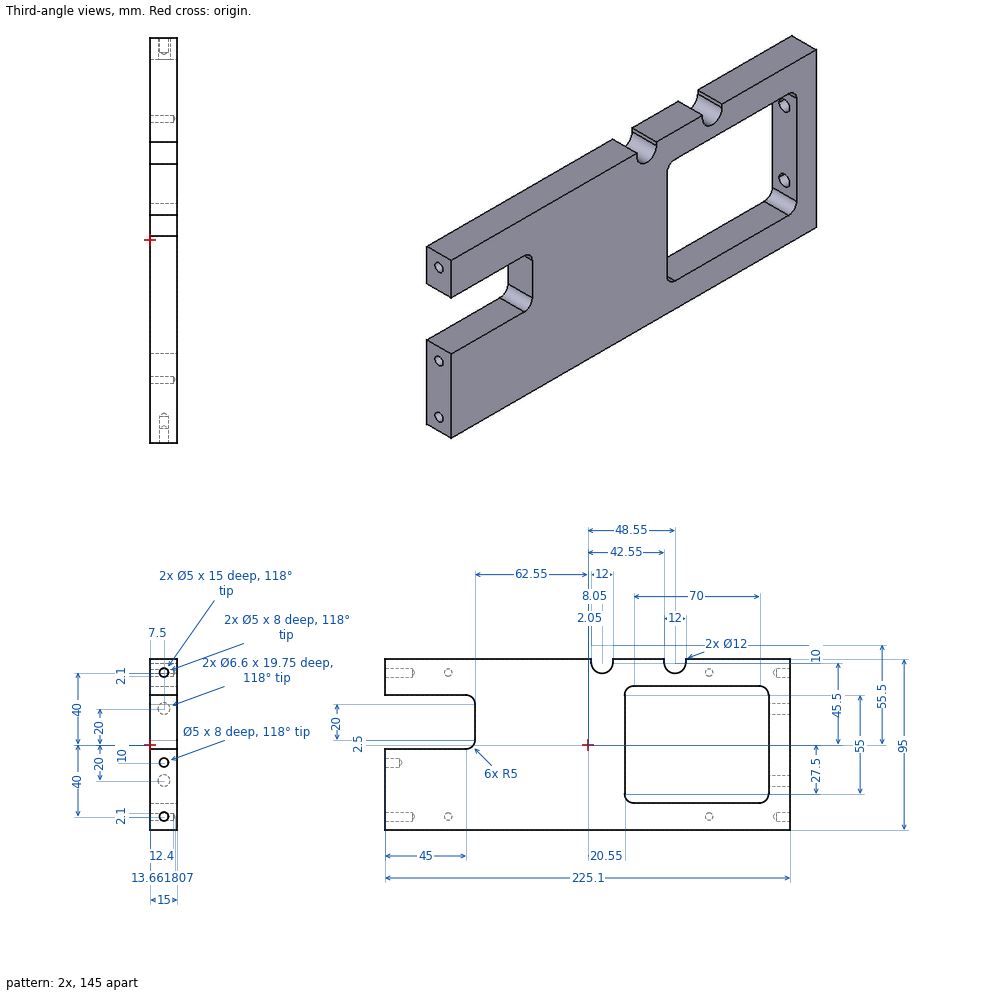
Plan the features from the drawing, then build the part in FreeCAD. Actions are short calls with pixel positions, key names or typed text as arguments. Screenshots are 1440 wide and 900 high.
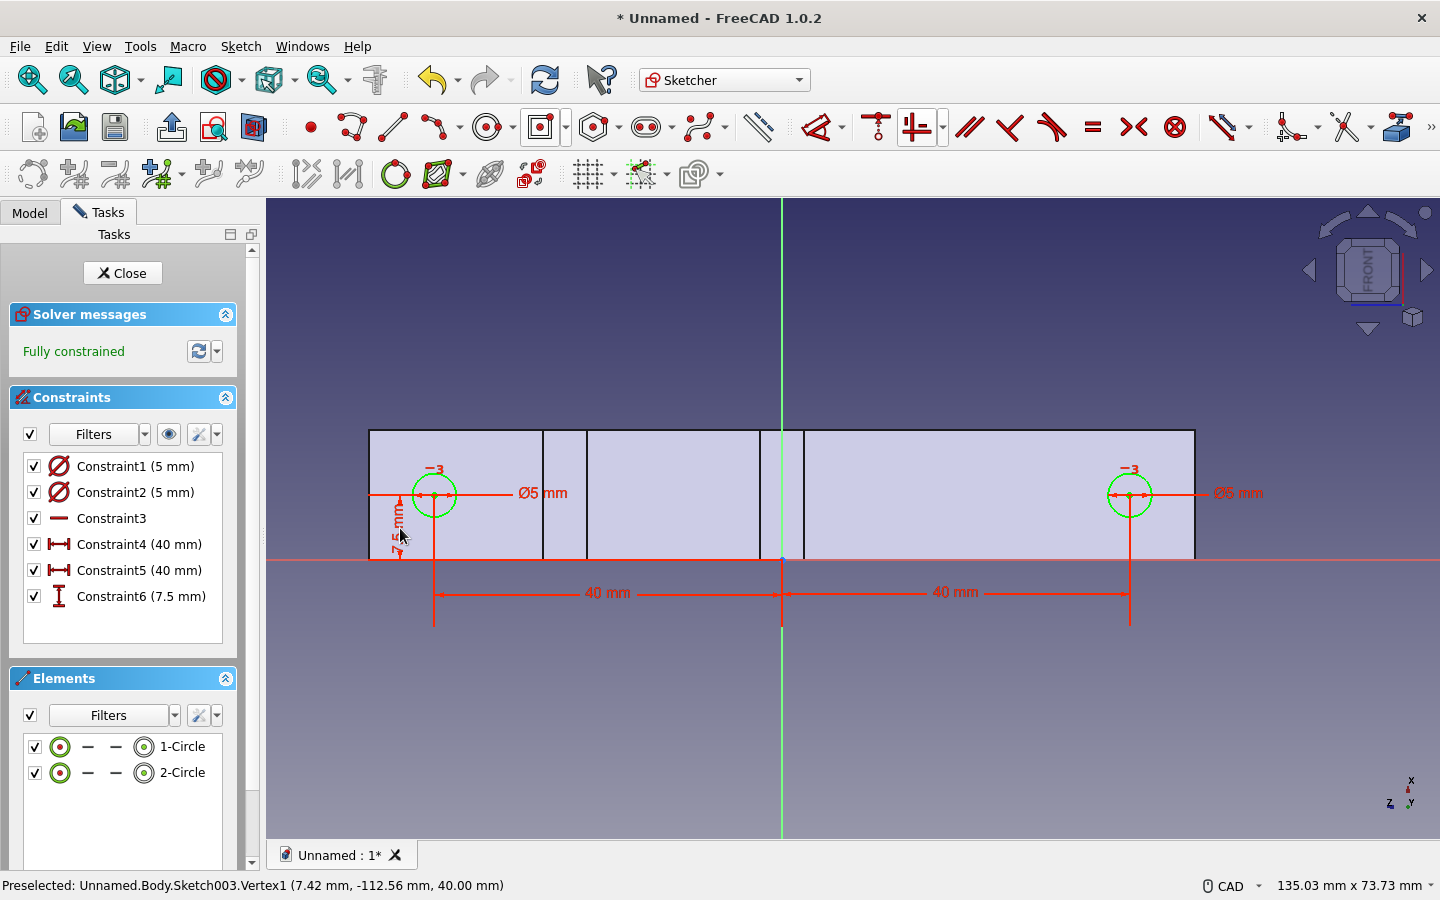
click(123, 273)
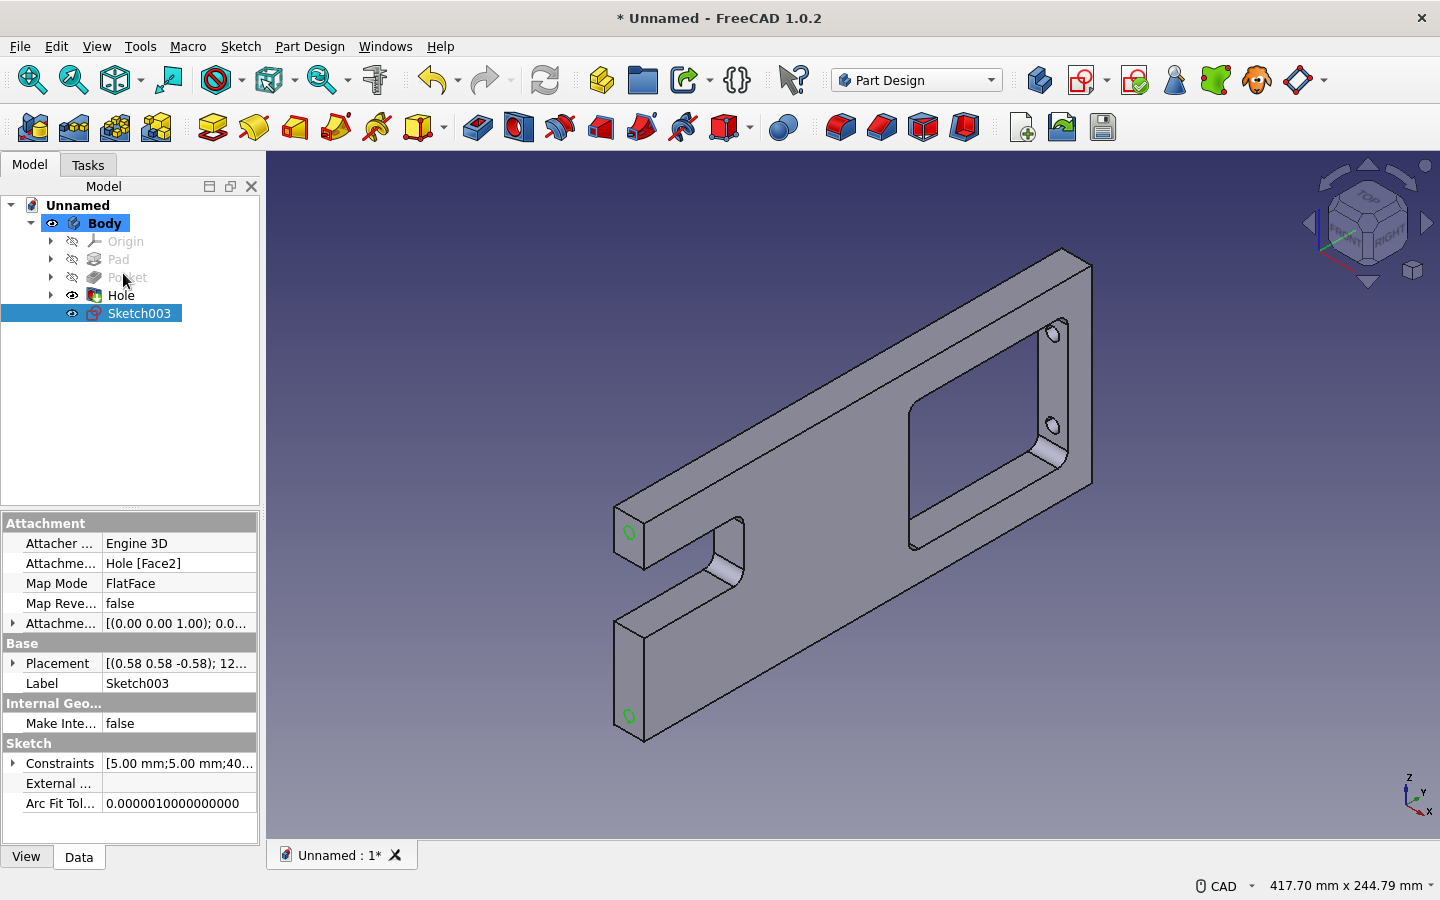
click(519, 128)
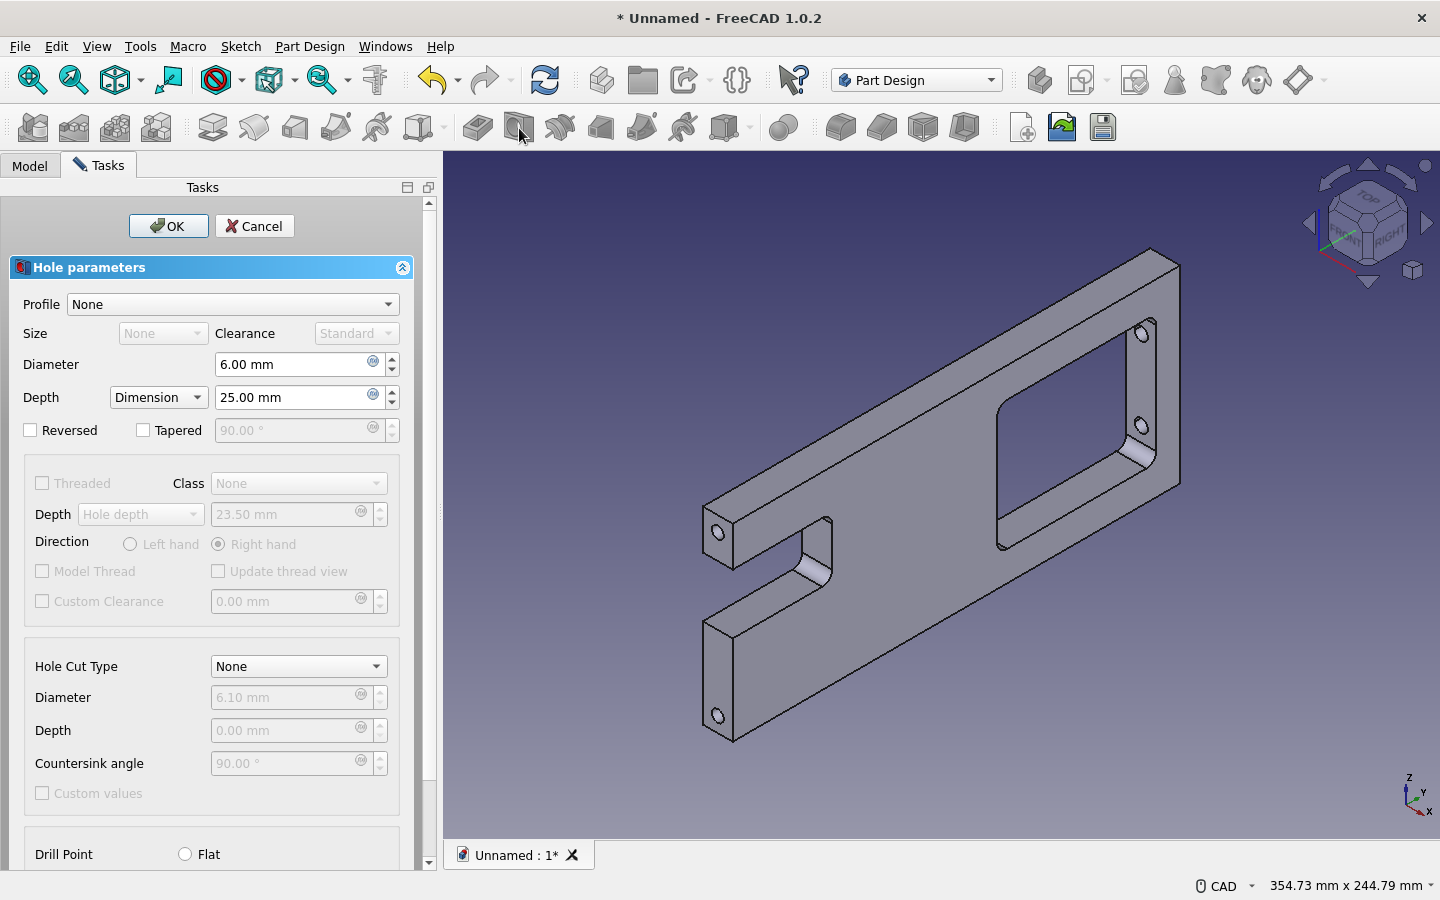
triple_click(300, 364)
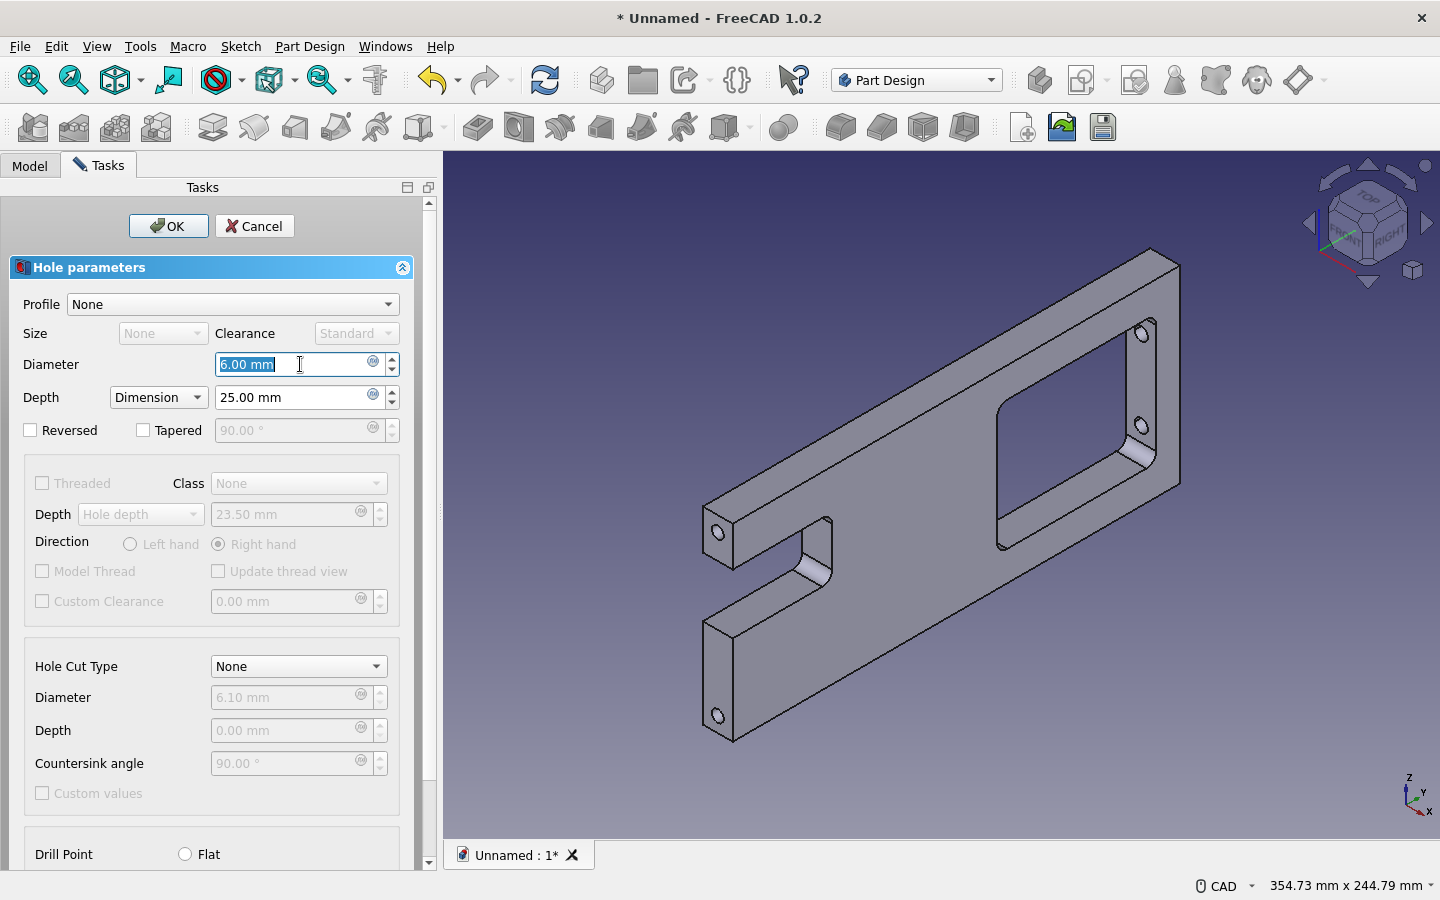
text(5)
key(Tab)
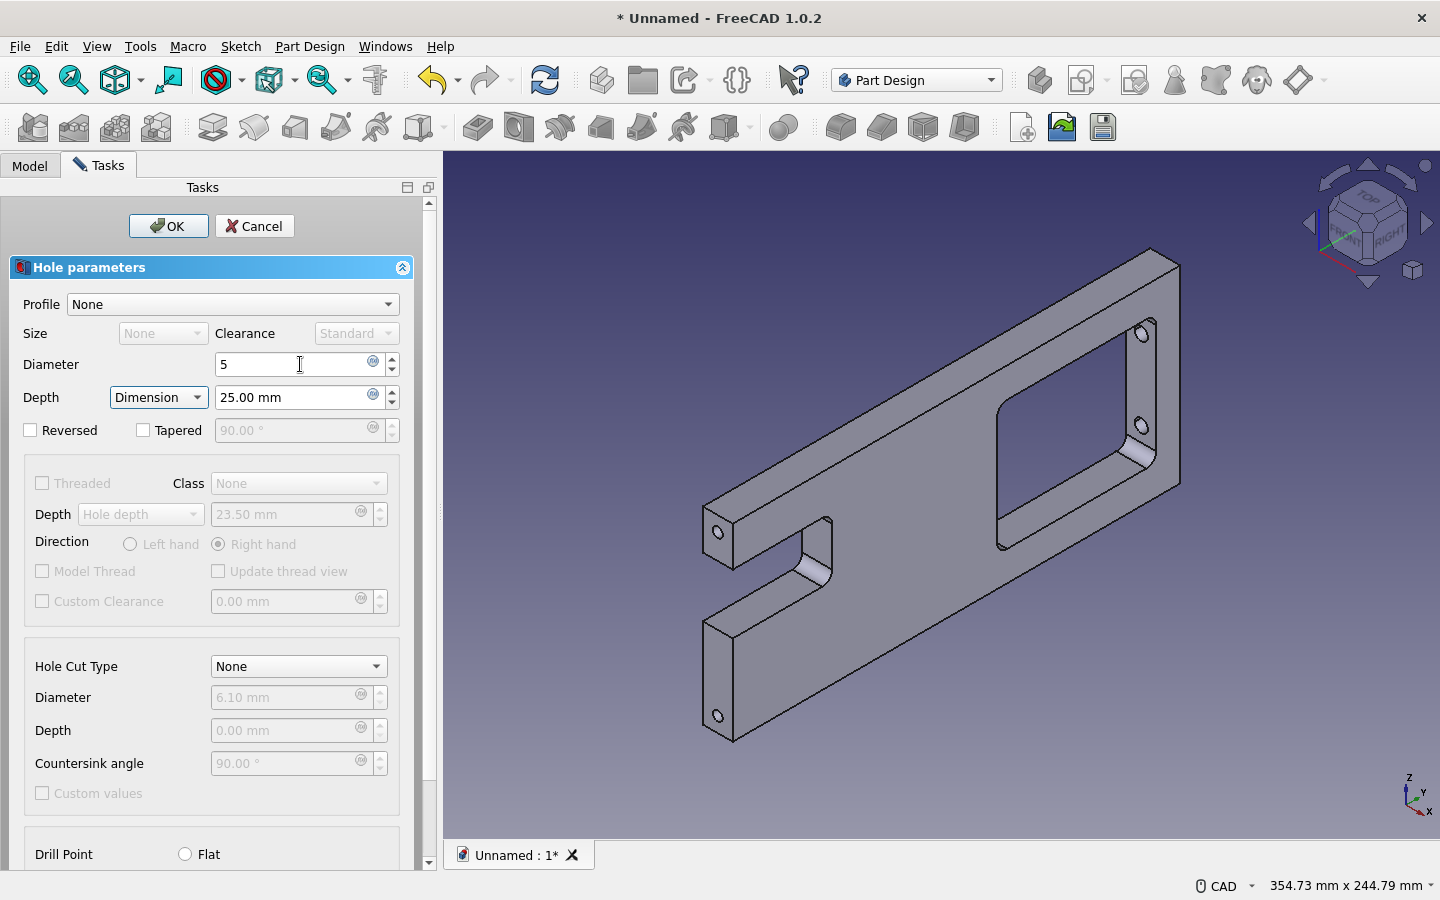
triple_click(300, 398)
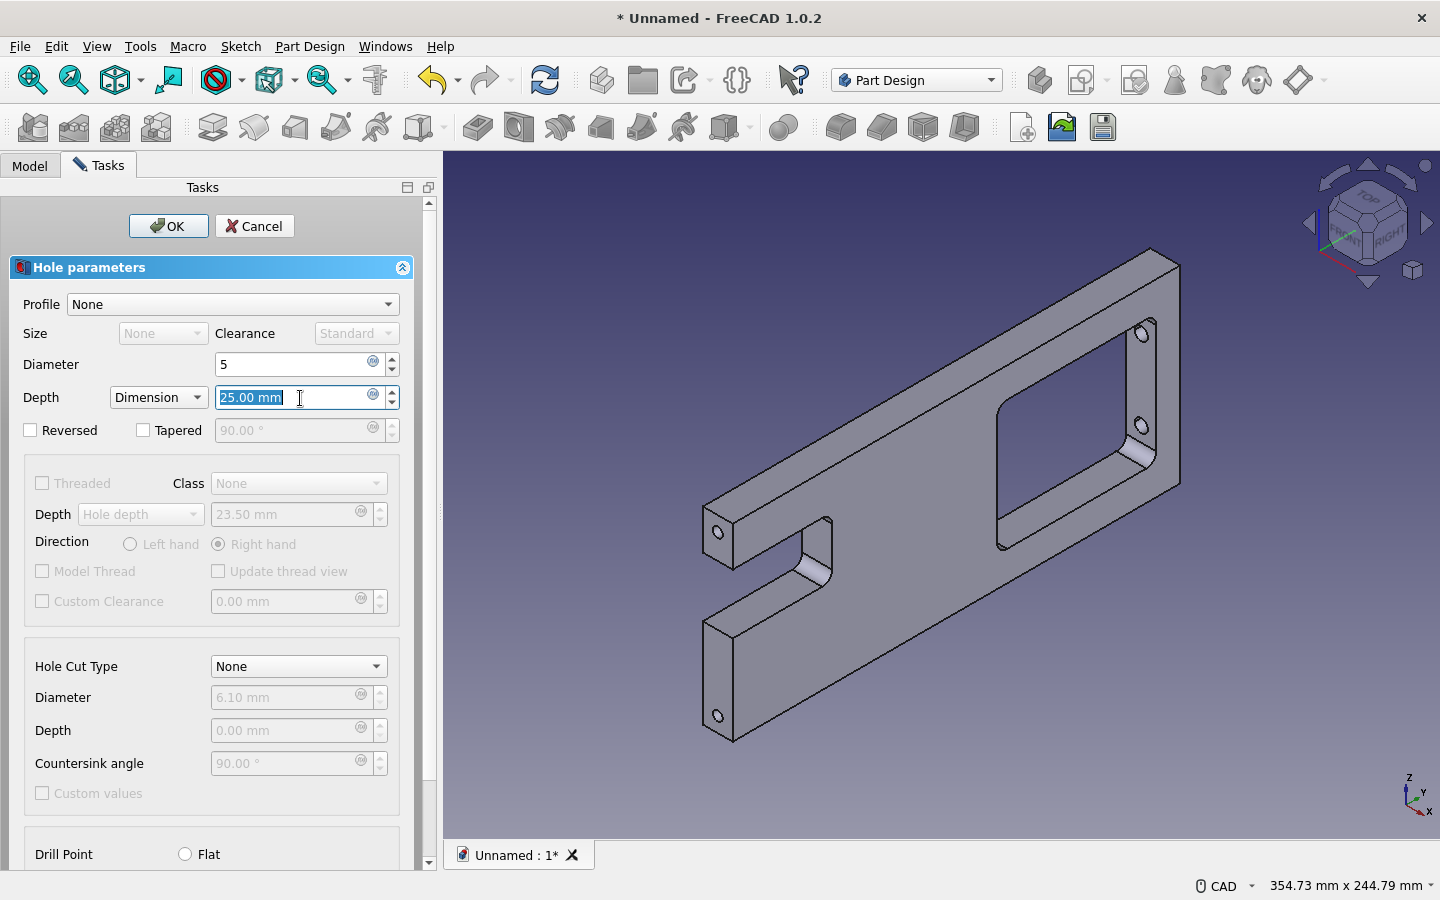
text(15)
key(Tab)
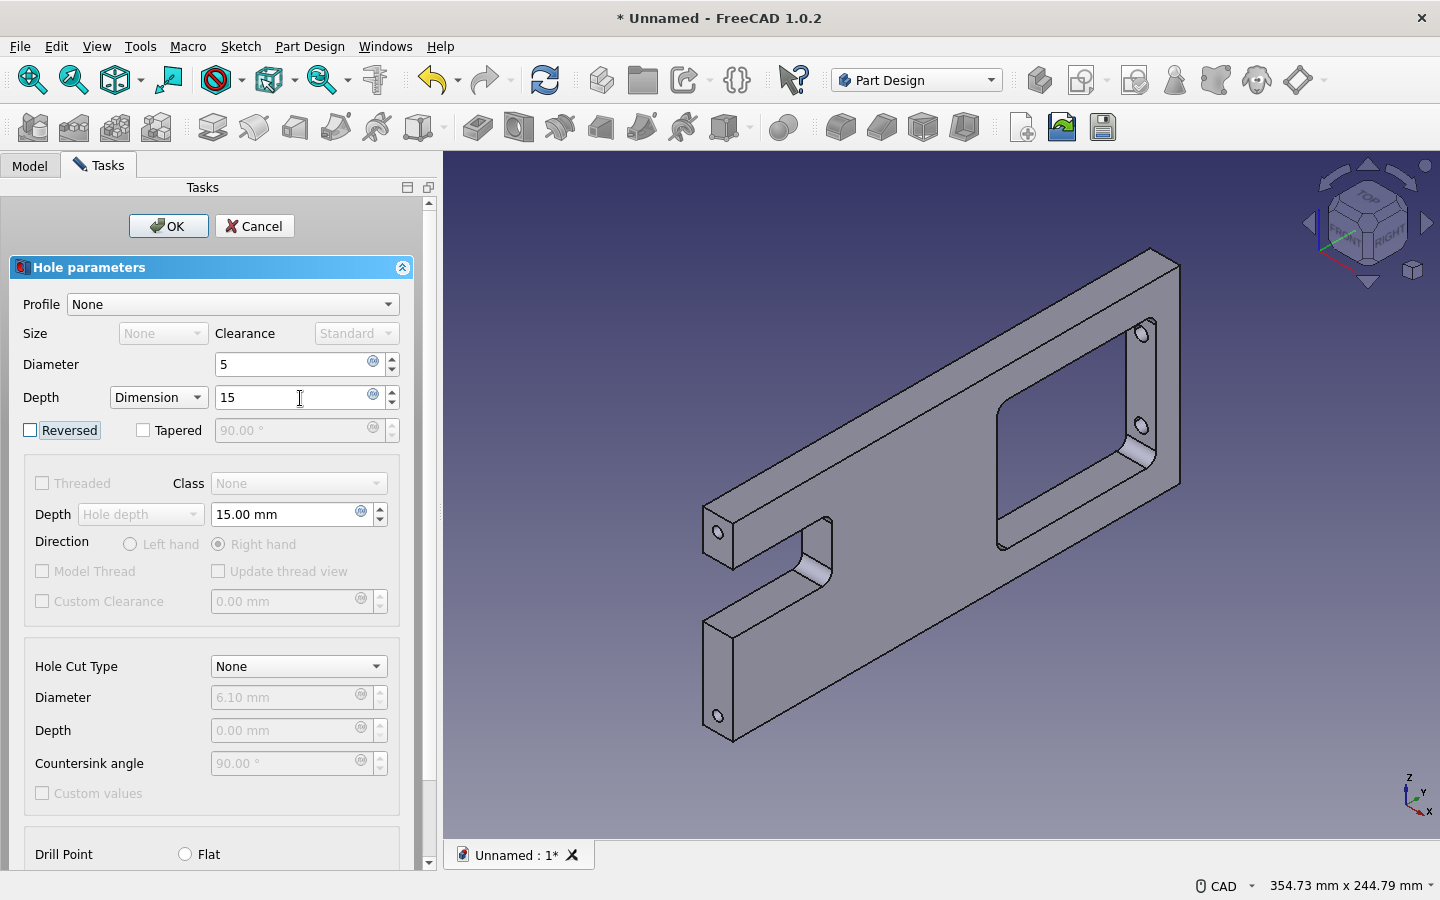
click(169, 226)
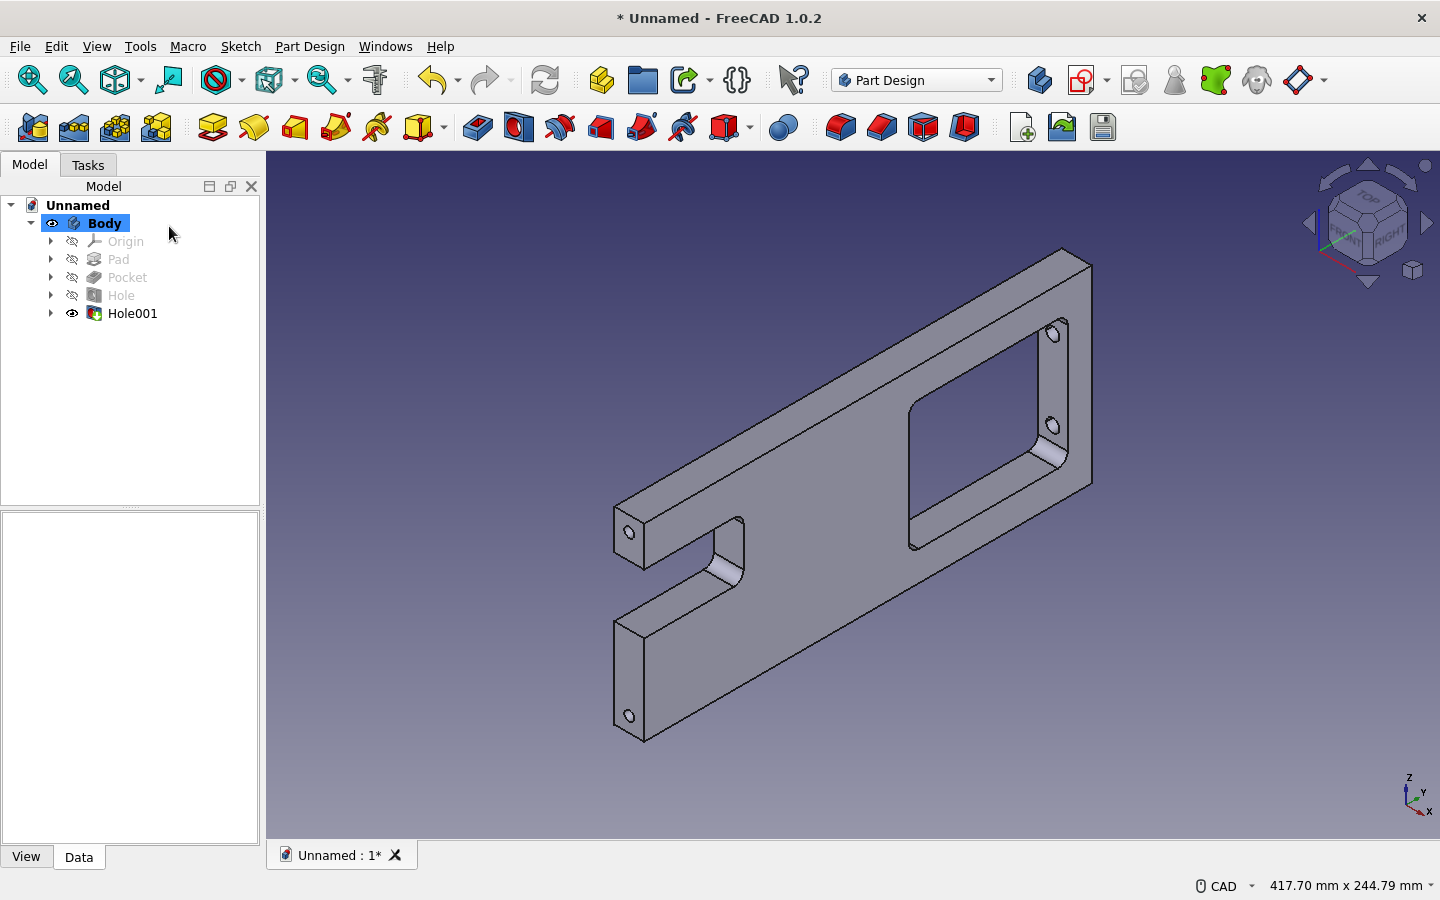
click(629, 666)